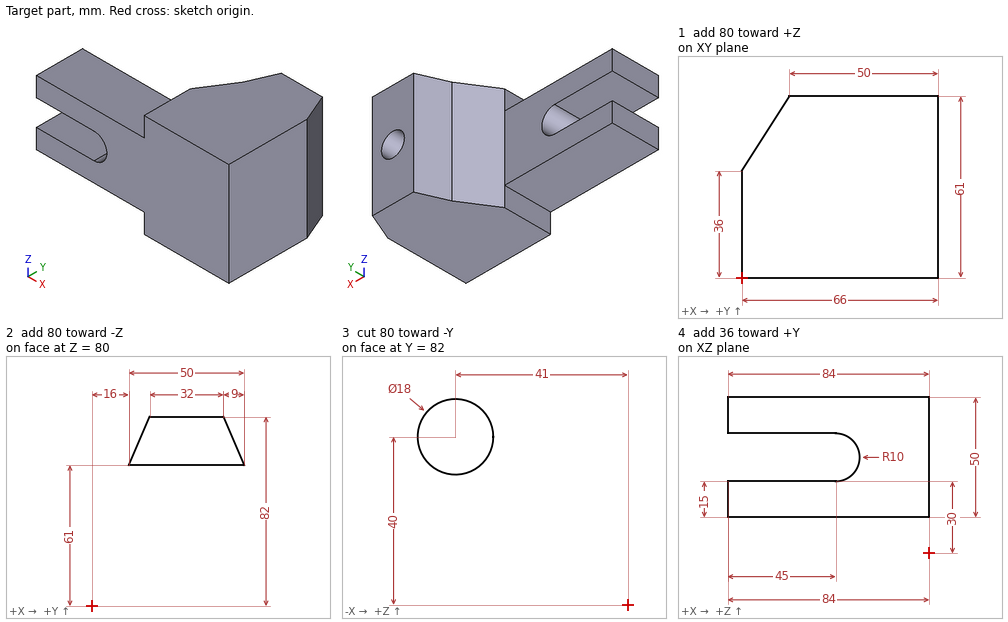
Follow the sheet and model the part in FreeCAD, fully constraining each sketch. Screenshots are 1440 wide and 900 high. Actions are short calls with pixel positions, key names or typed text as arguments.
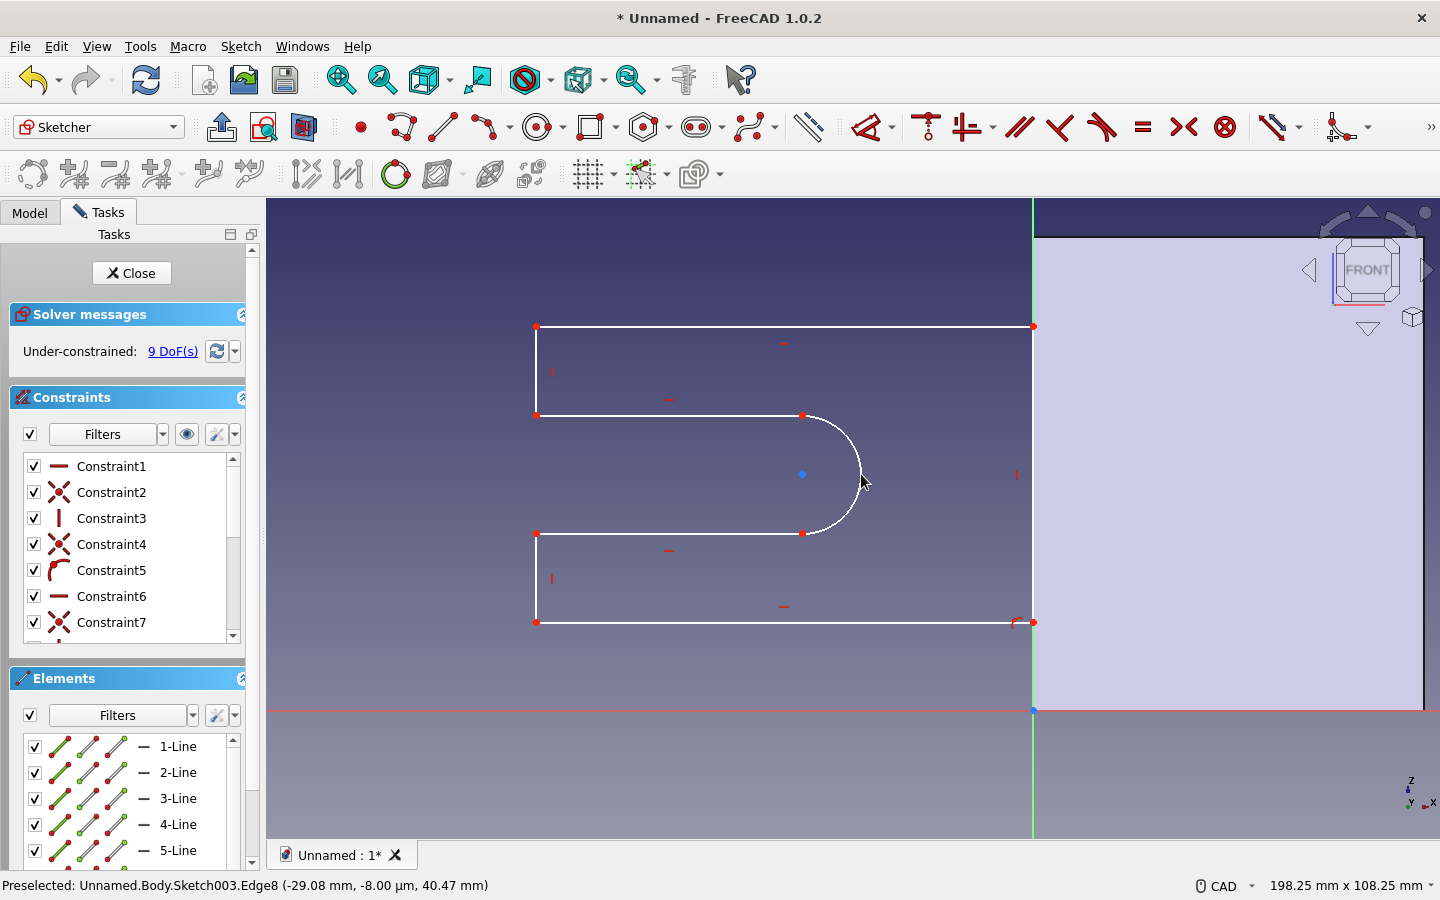
click(722, 534)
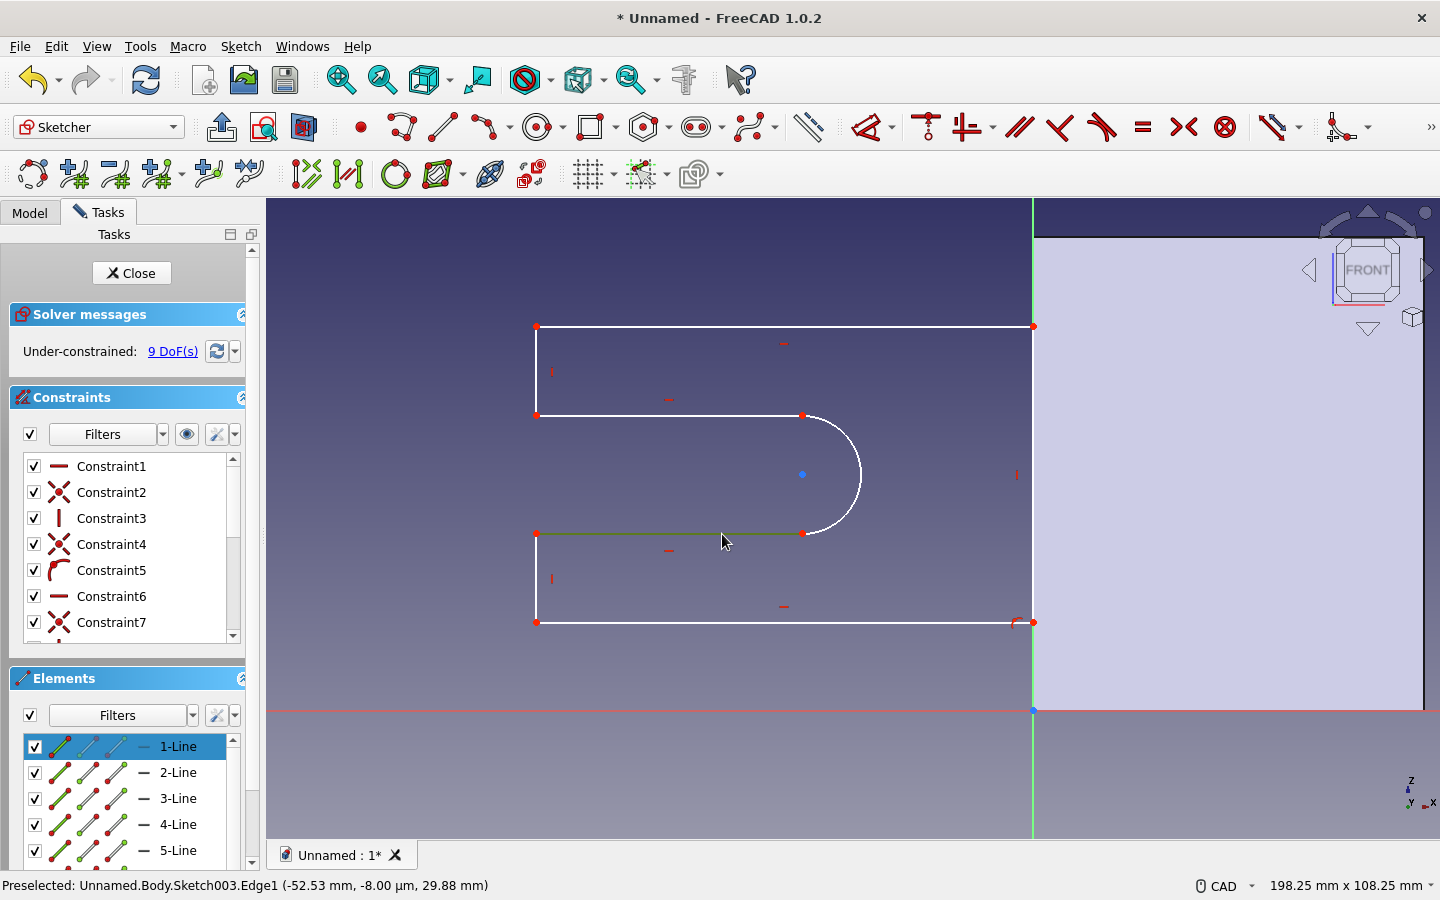
click(850, 510)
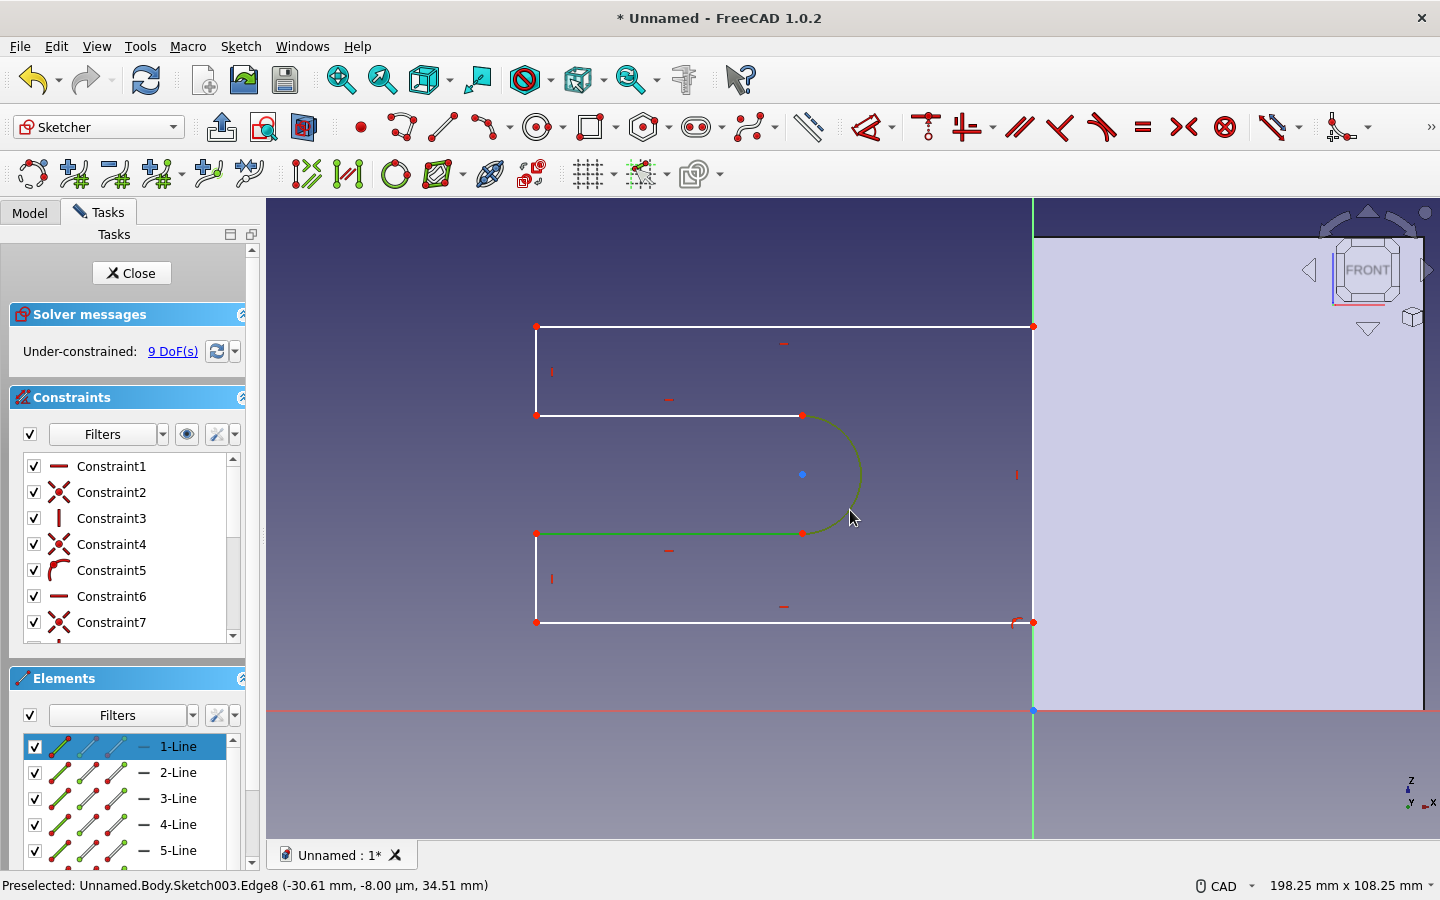
key(t)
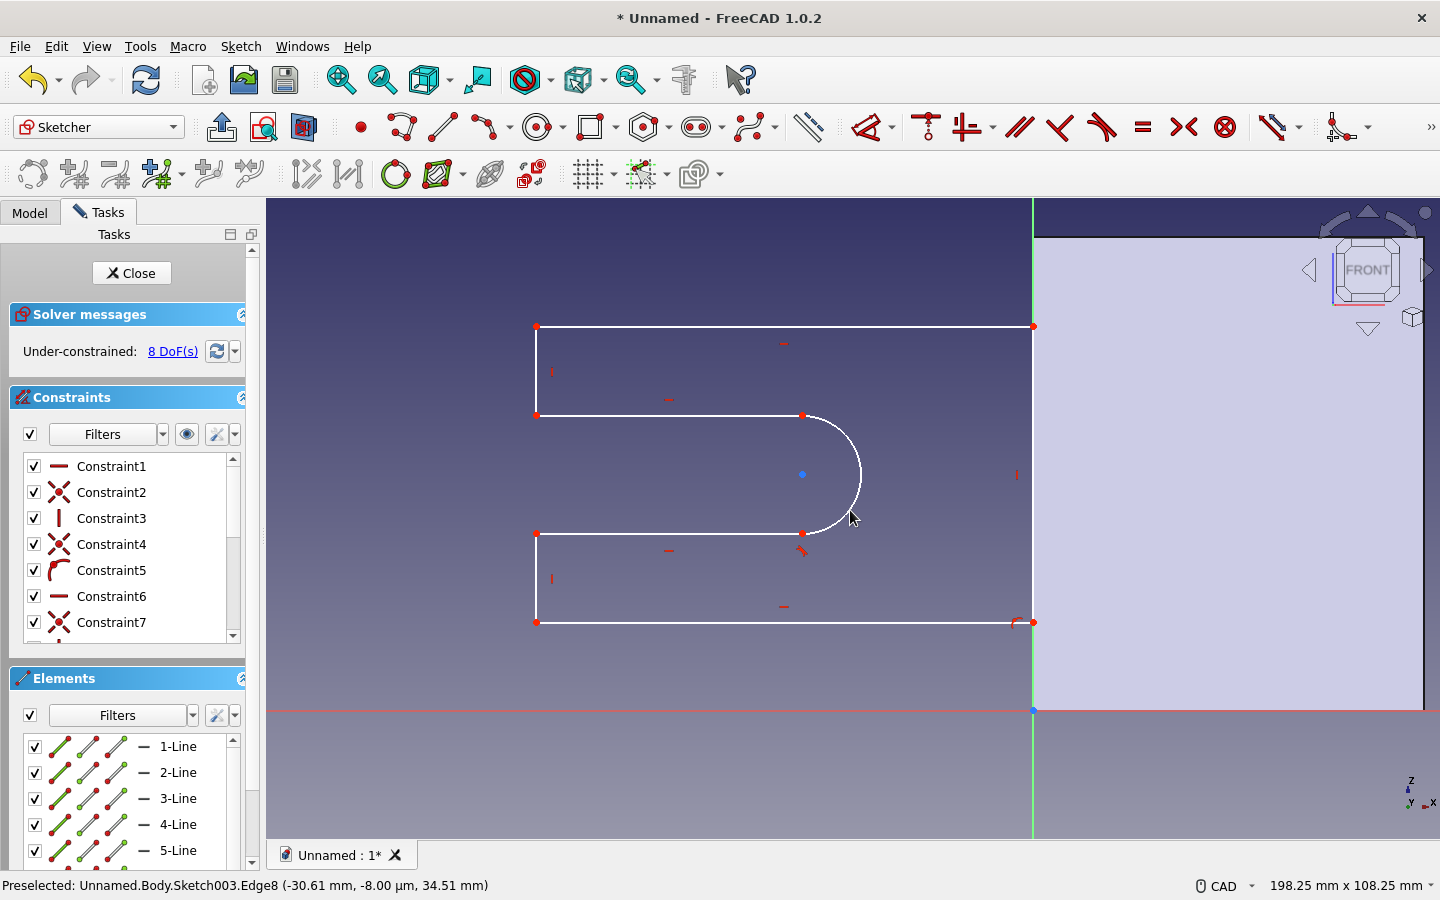
click(616, 416)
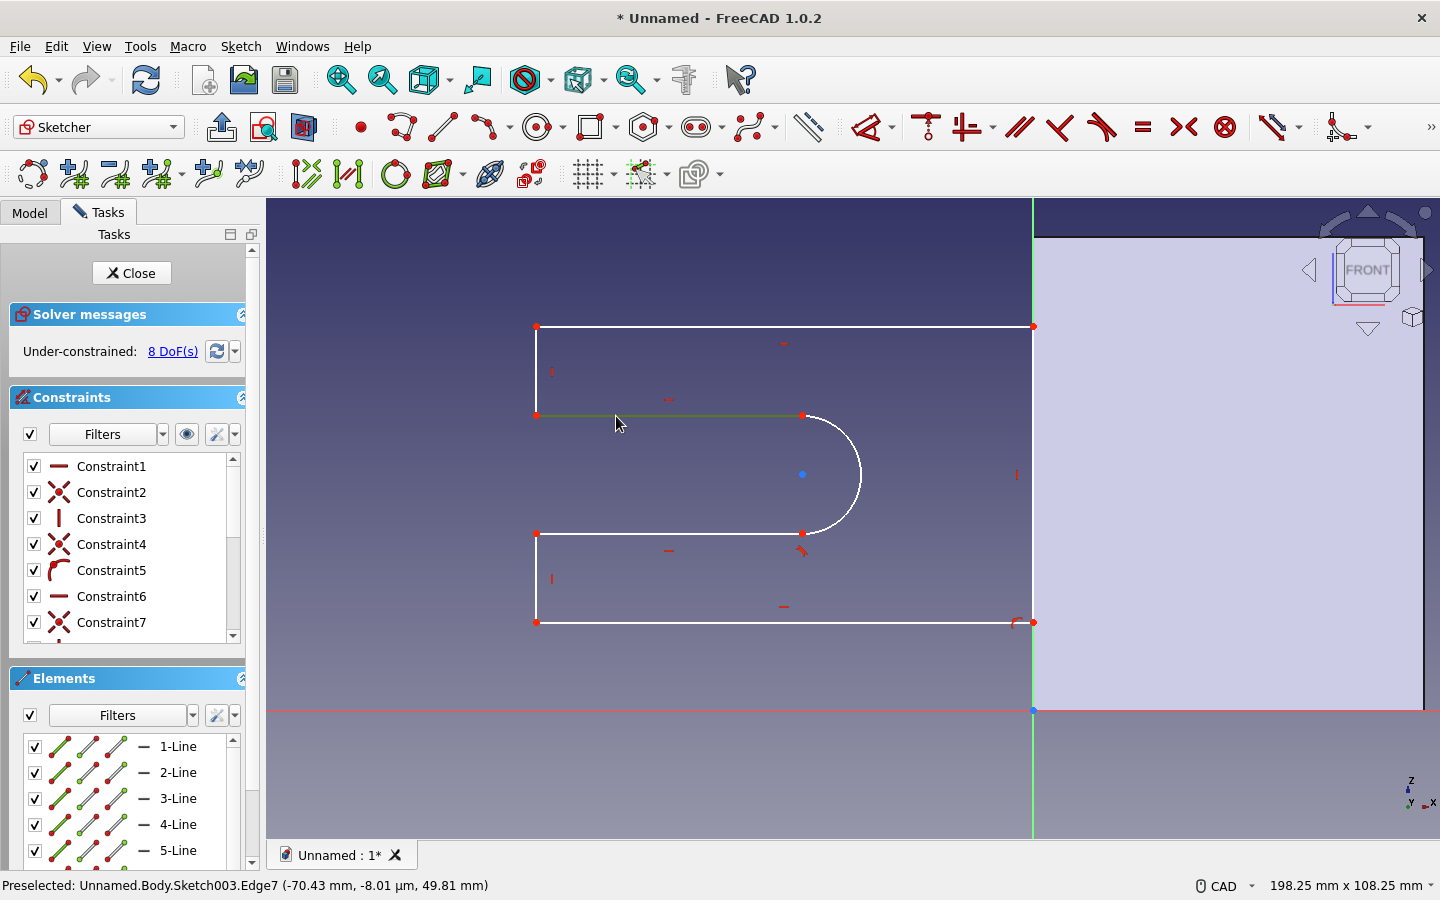
click(850, 510)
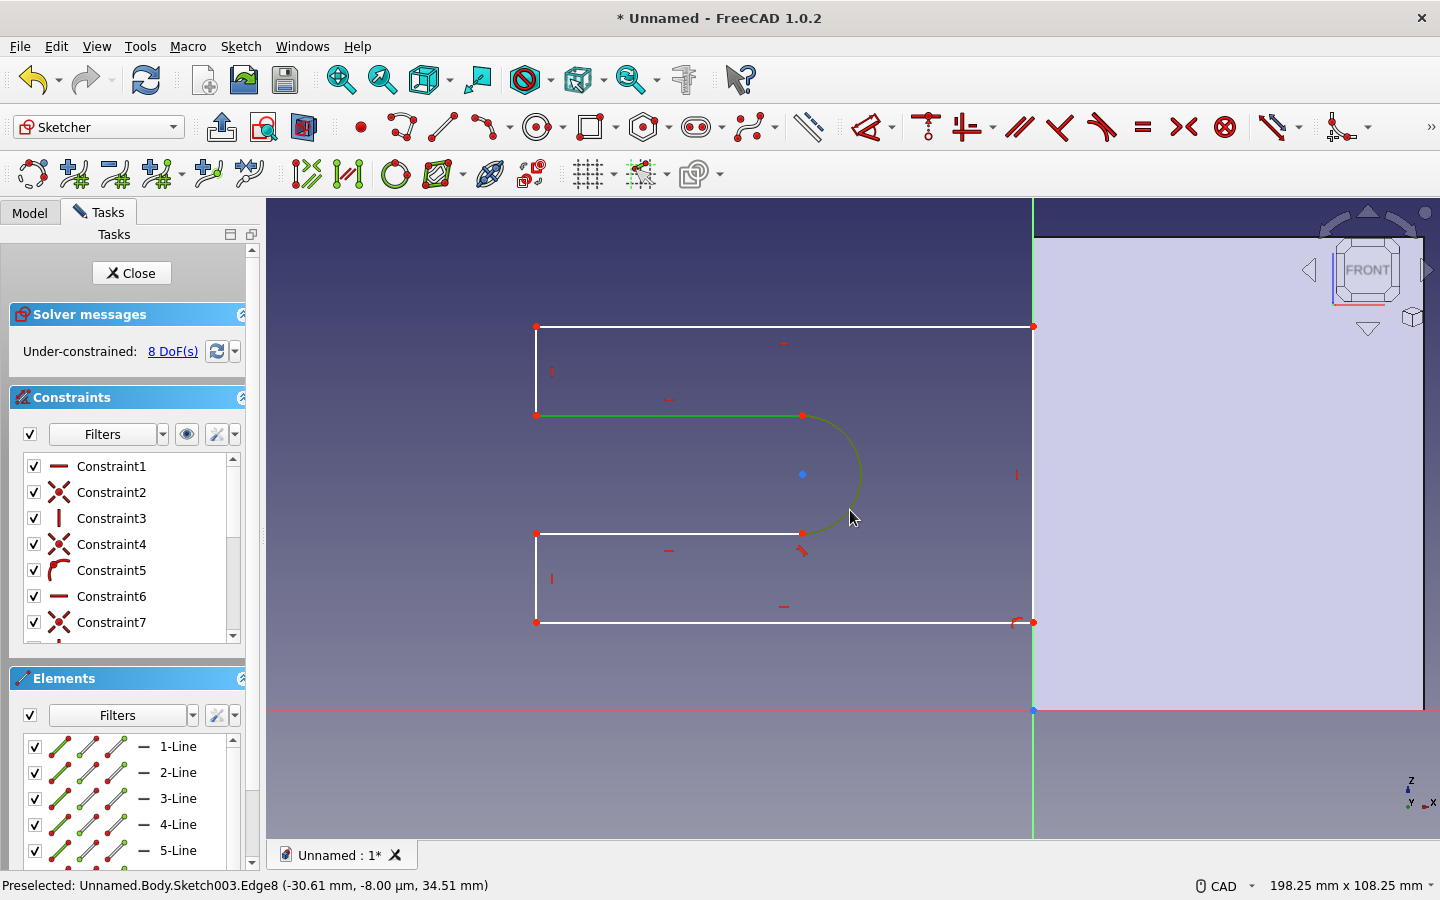
key(t)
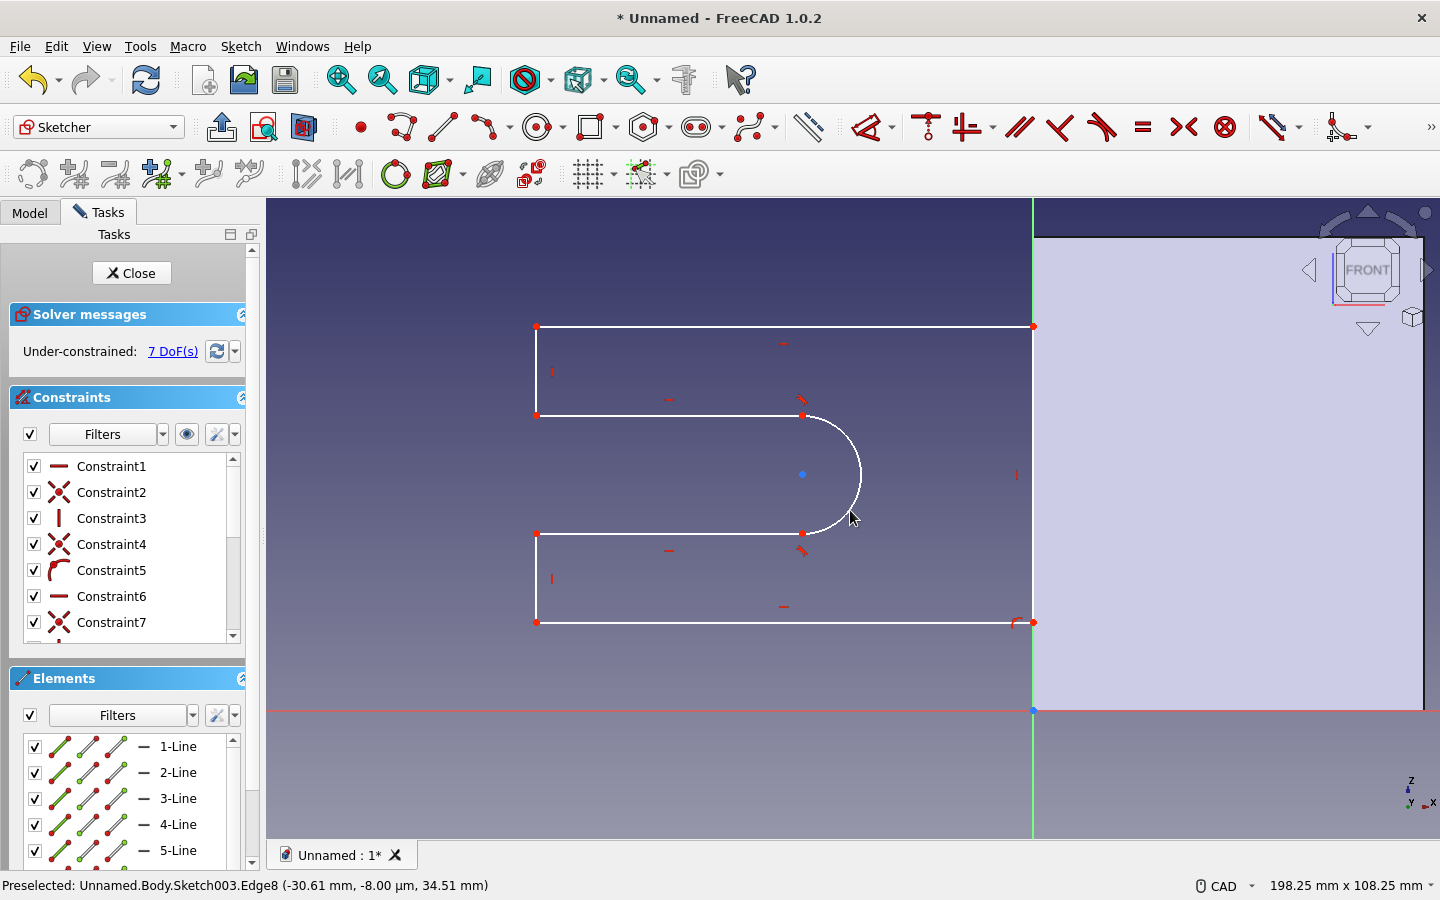
key(d)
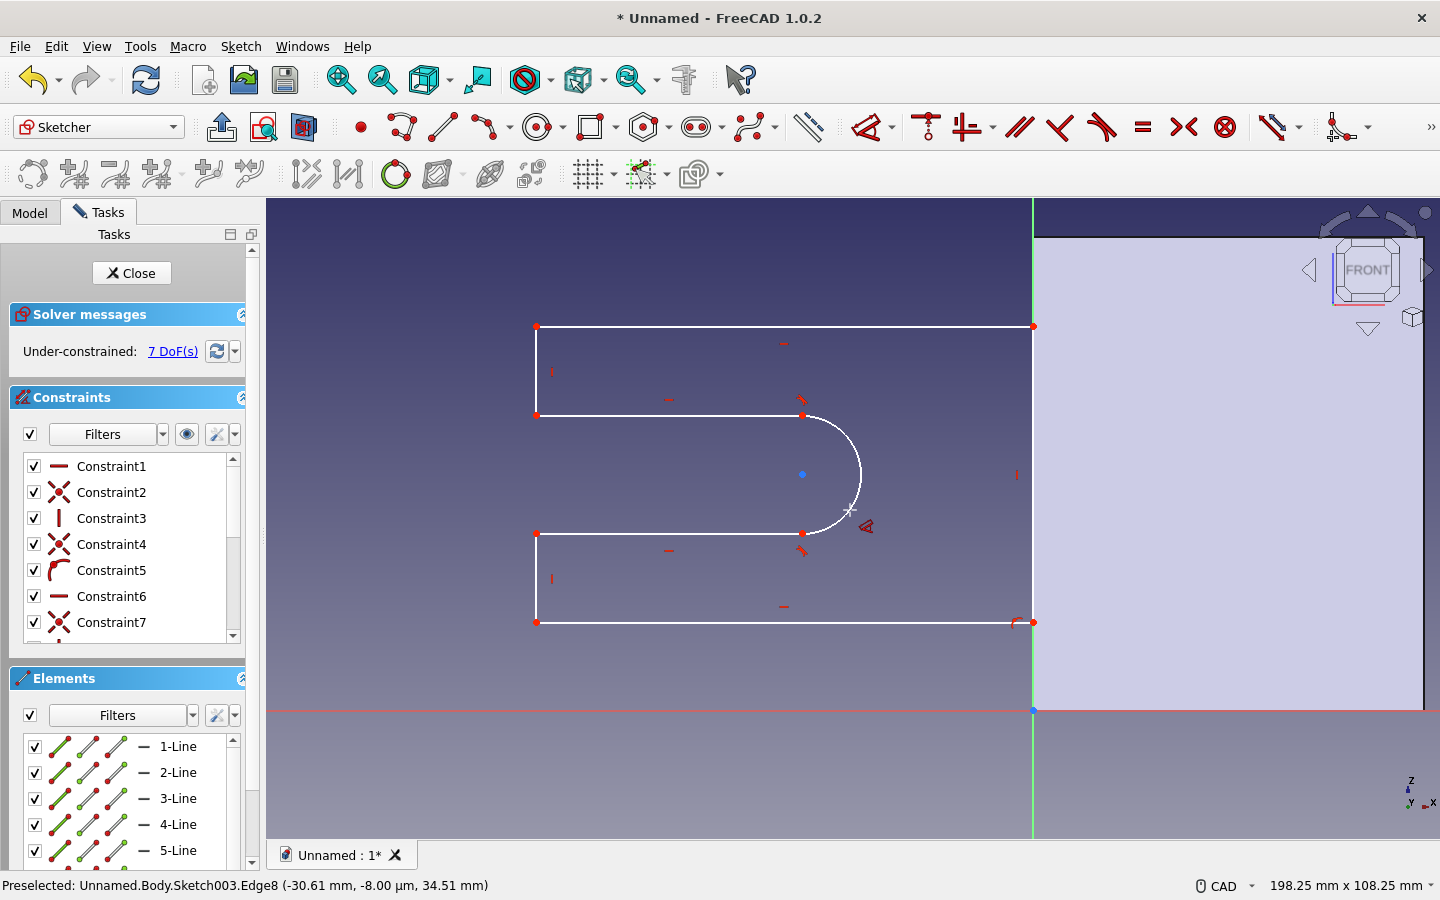
click(850, 510)
click(876, 529)